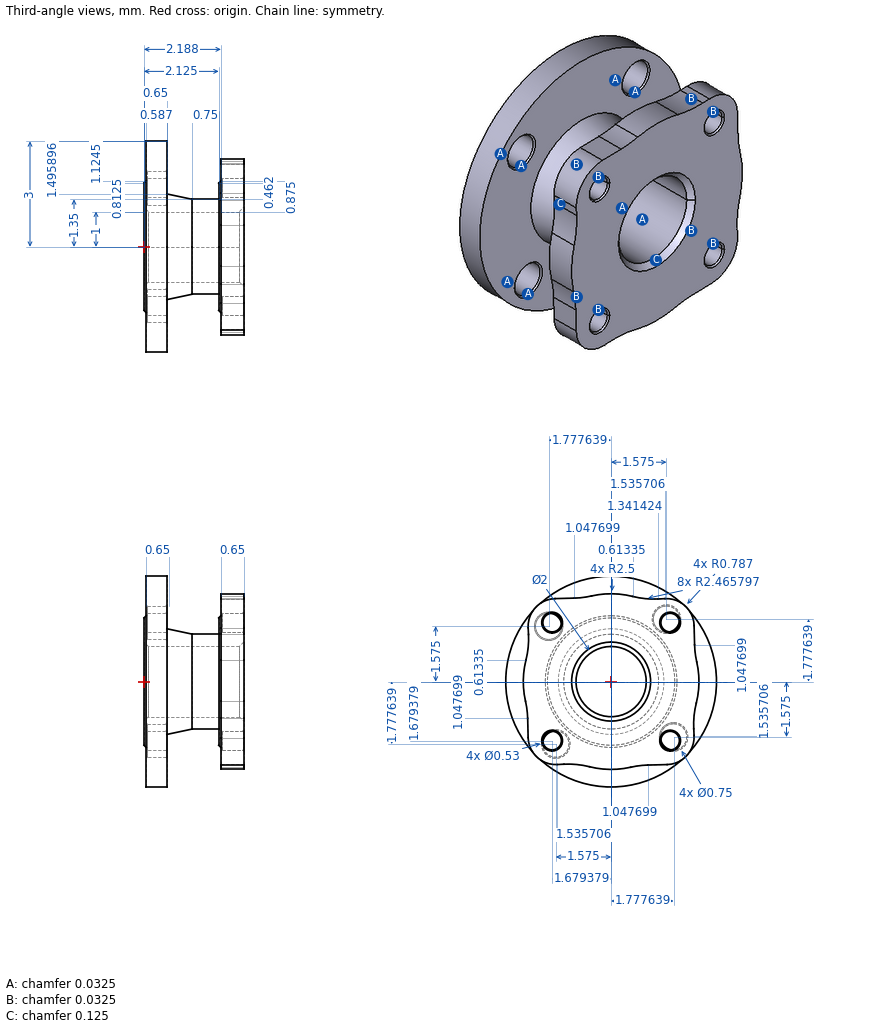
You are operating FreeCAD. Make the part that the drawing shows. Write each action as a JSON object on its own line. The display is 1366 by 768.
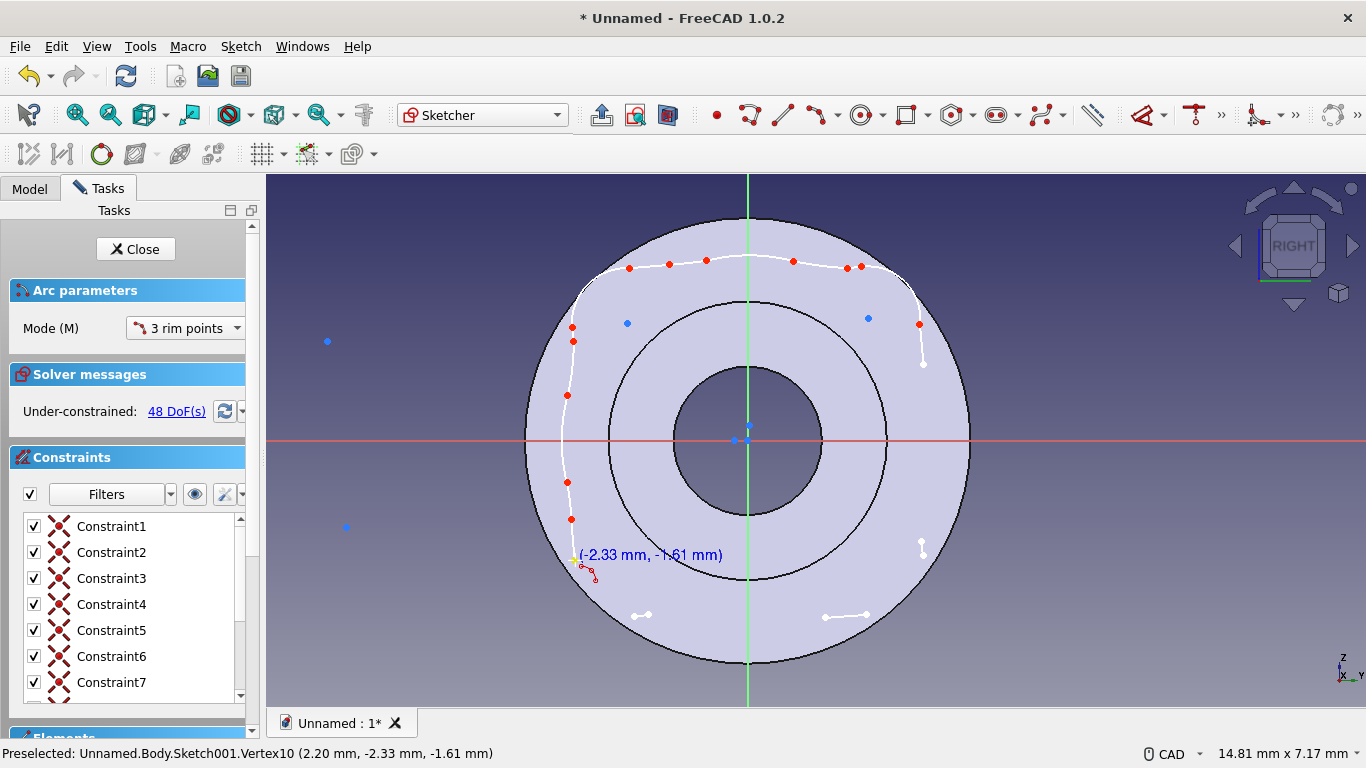
{"action": "scroll", "coordinate": [634, 616], "scroll_direction": "up", "scroll_amount": 4}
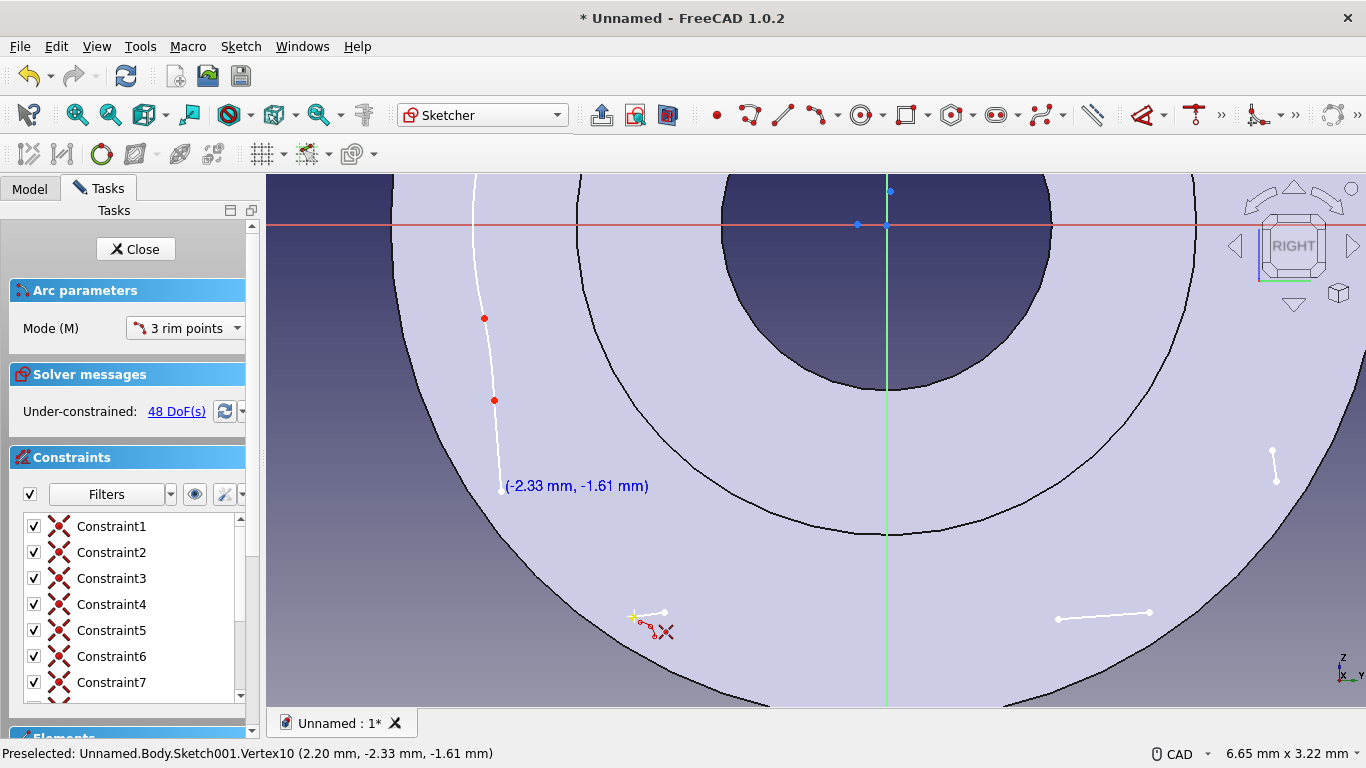
{"action": "left_click", "coordinate": [634, 617]}
{"action": "left_click", "coordinate": [538, 581]}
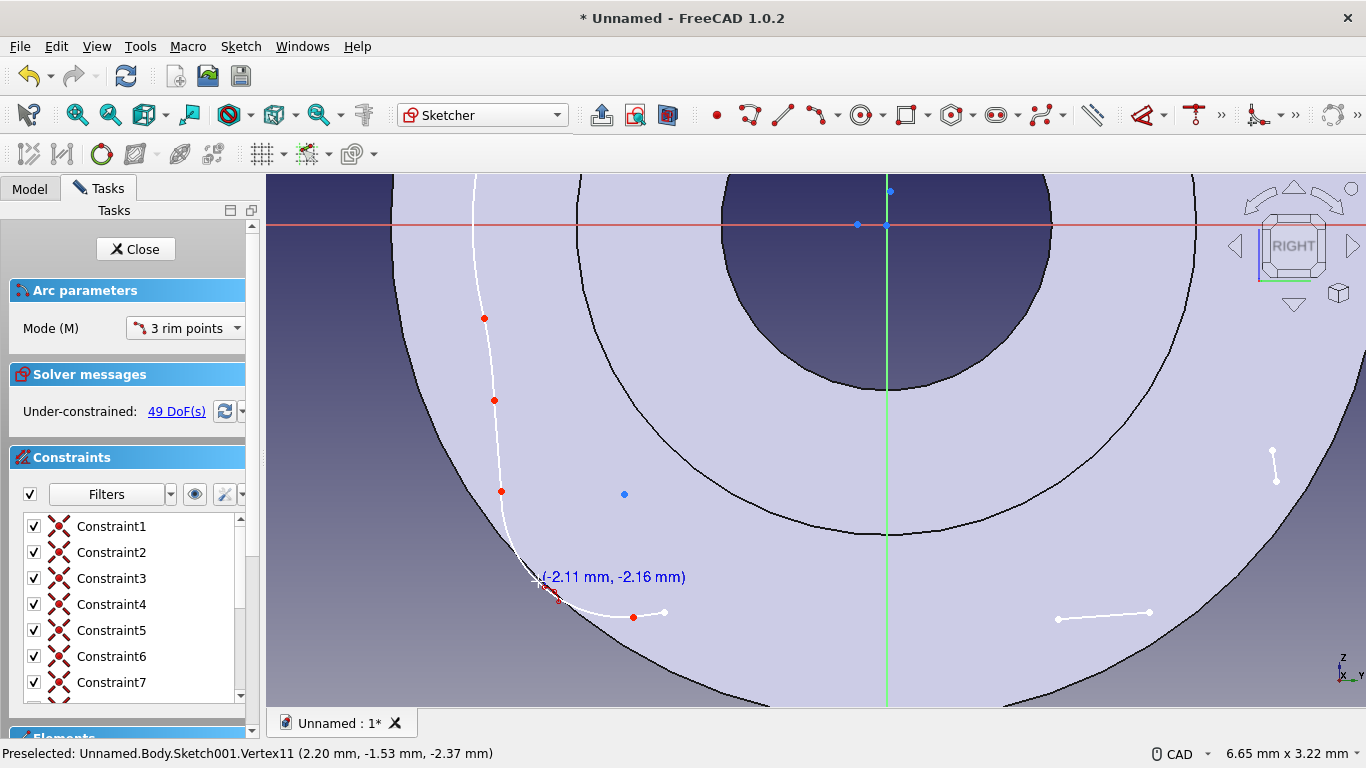
{"action": "left_click", "coordinate": [665, 613]}
{"action": "left_click", "coordinate": [785, 626]}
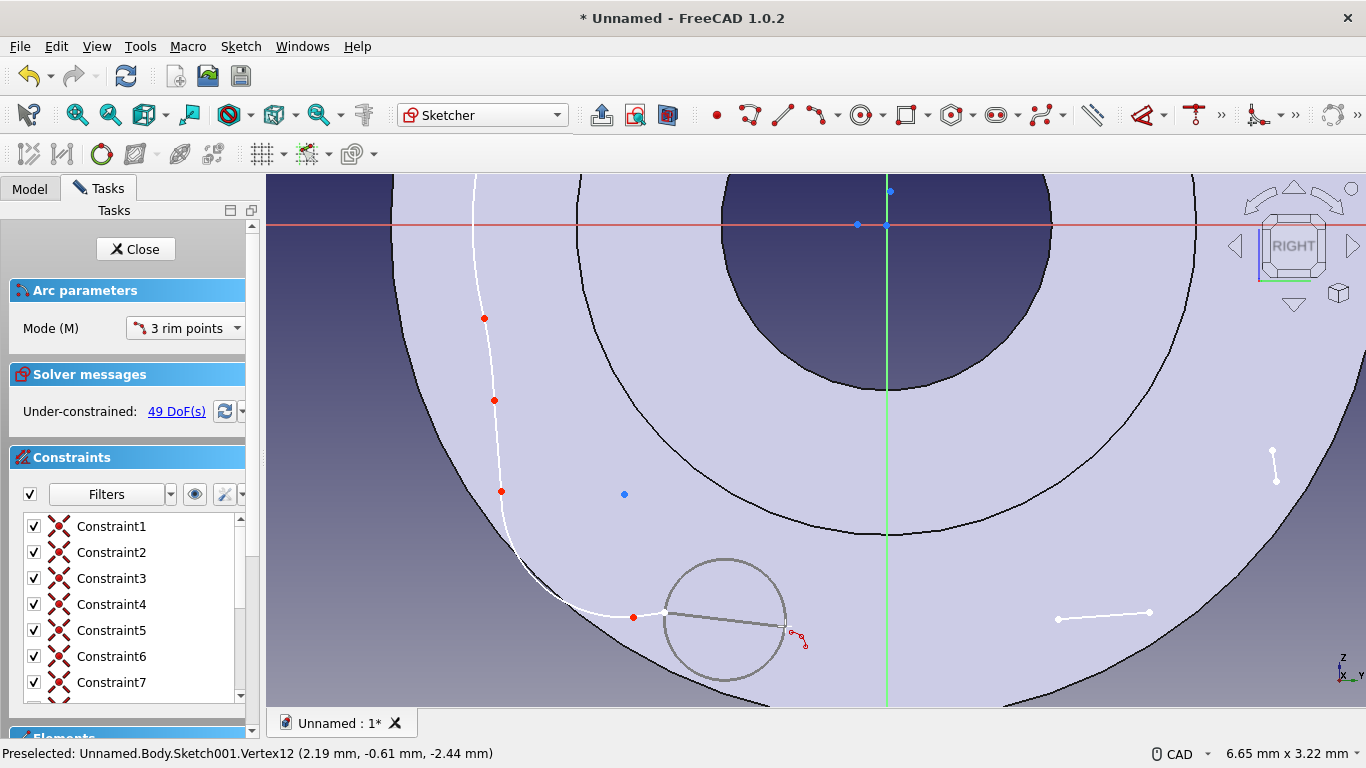
{"action": "scroll", "coordinate": [725, 615], "scroll_direction": "up", "scroll_amount": 7}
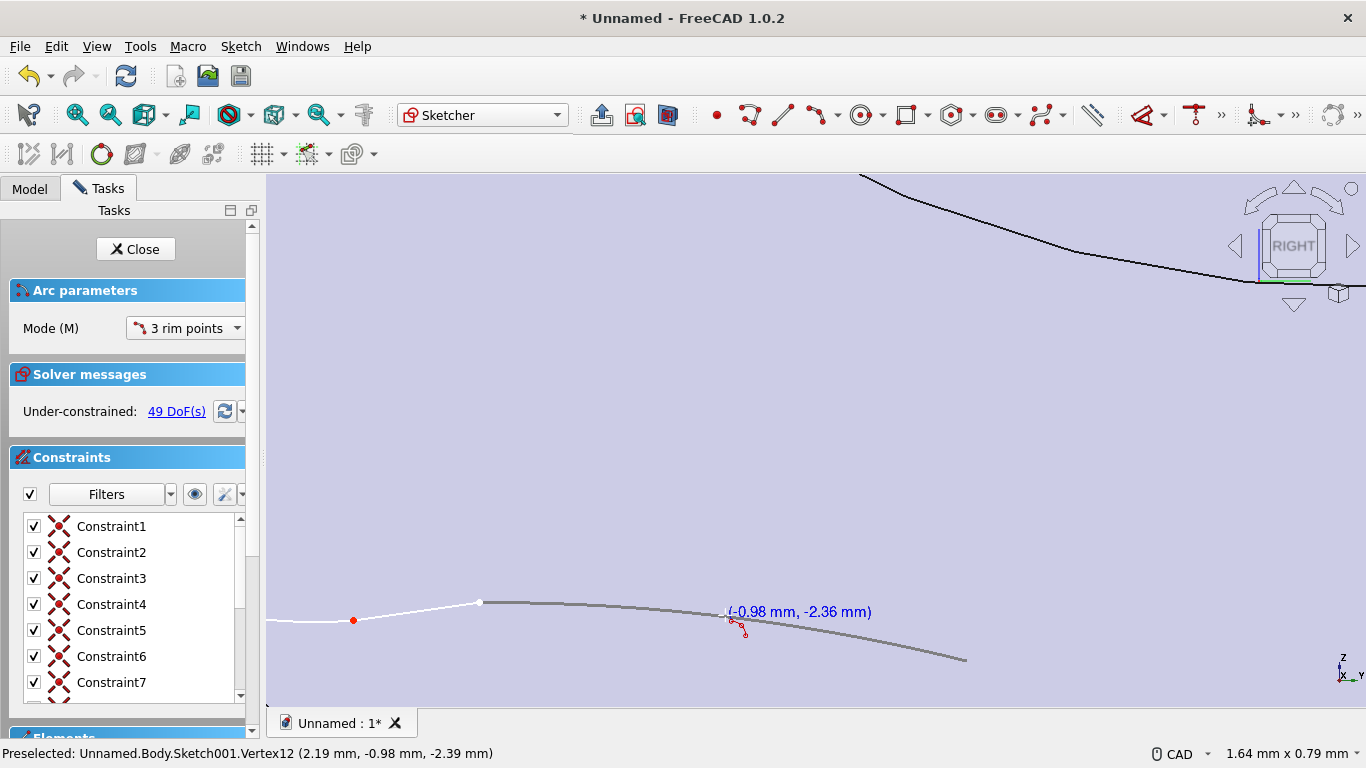
{"action": "left_click", "coordinate": [725, 614]}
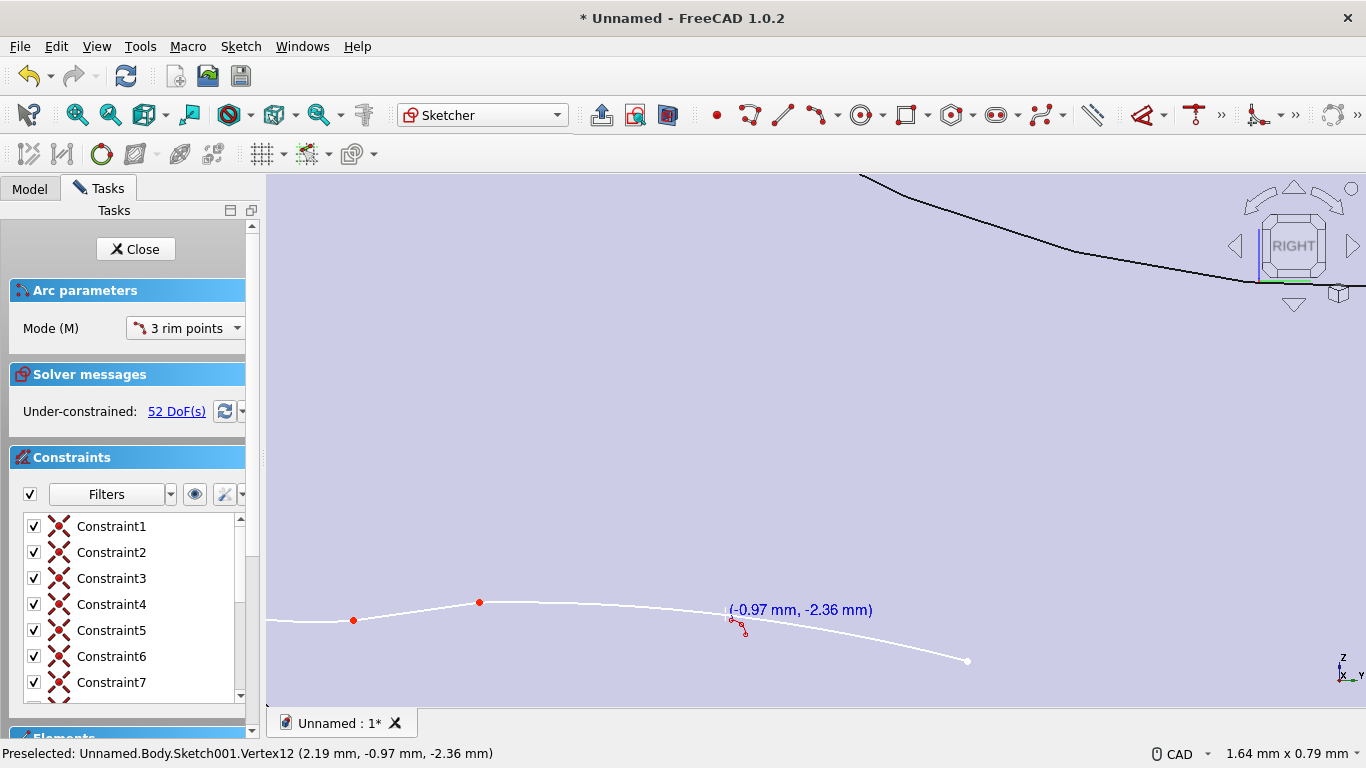
{"action": "scroll", "coordinate": [669, 616], "scroll_direction": "down", "scroll_amount": 11}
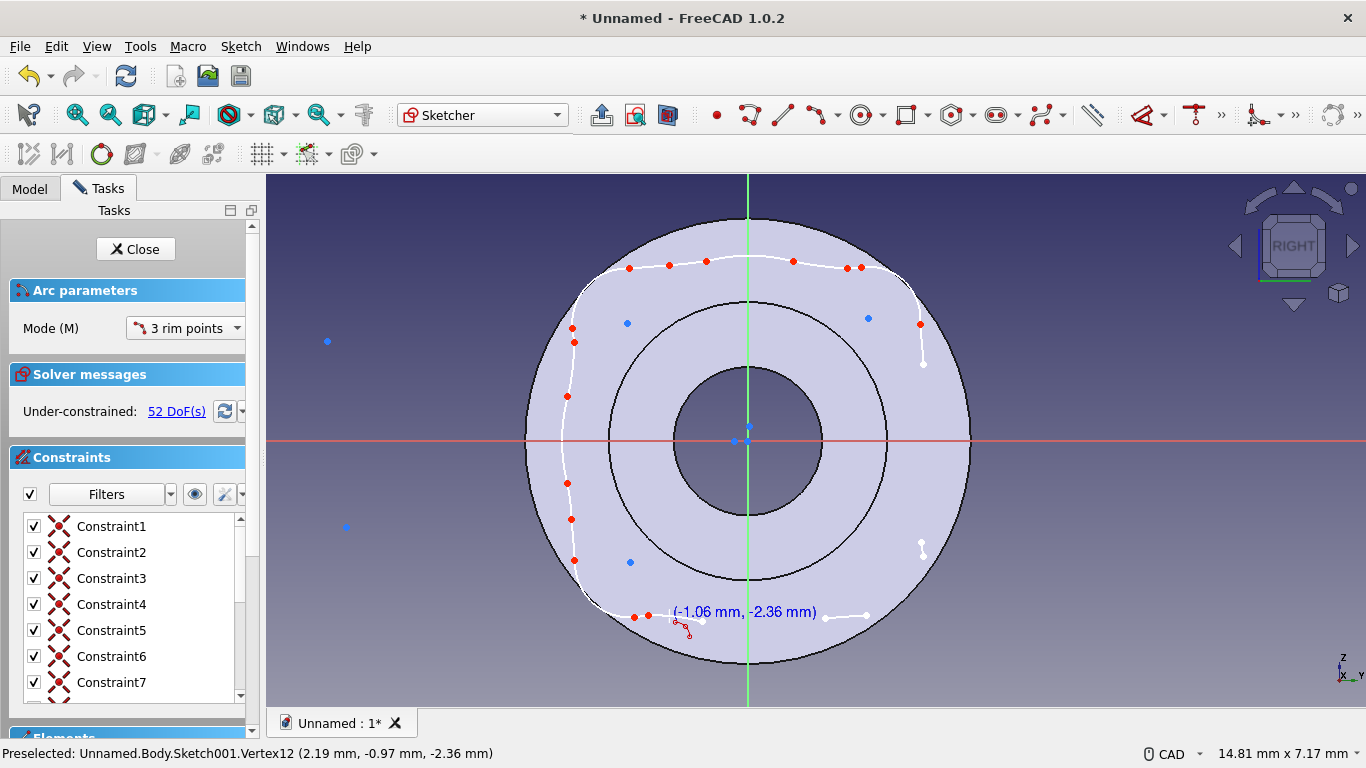
{"action": "left_click", "coordinate": [702, 622]}
{"action": "left_click", "coordinate": [789, 622]}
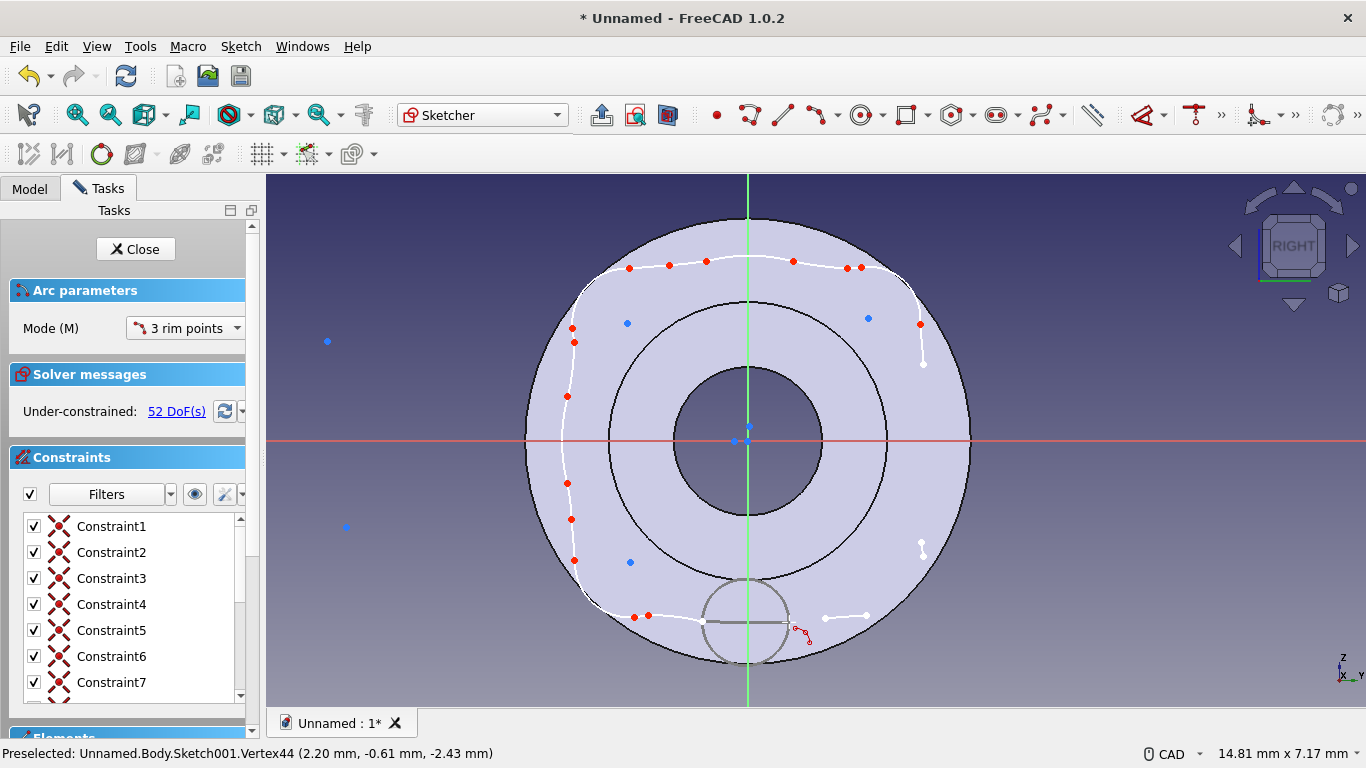
{"action": "scroll", "coordinate": [755, 627], "scroll_direction": "up", "scroll_amount": 6}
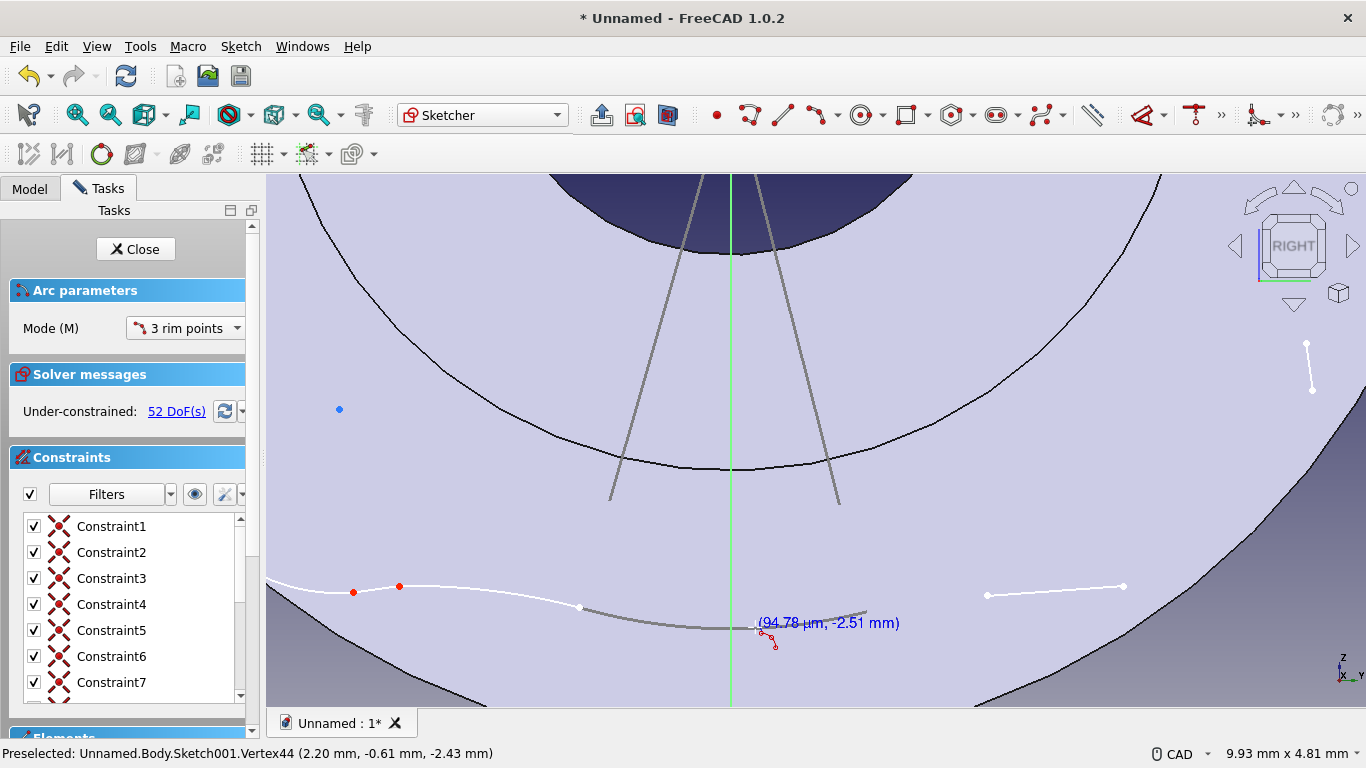
{"action": "left_click", "coordinate": [753, 624]}